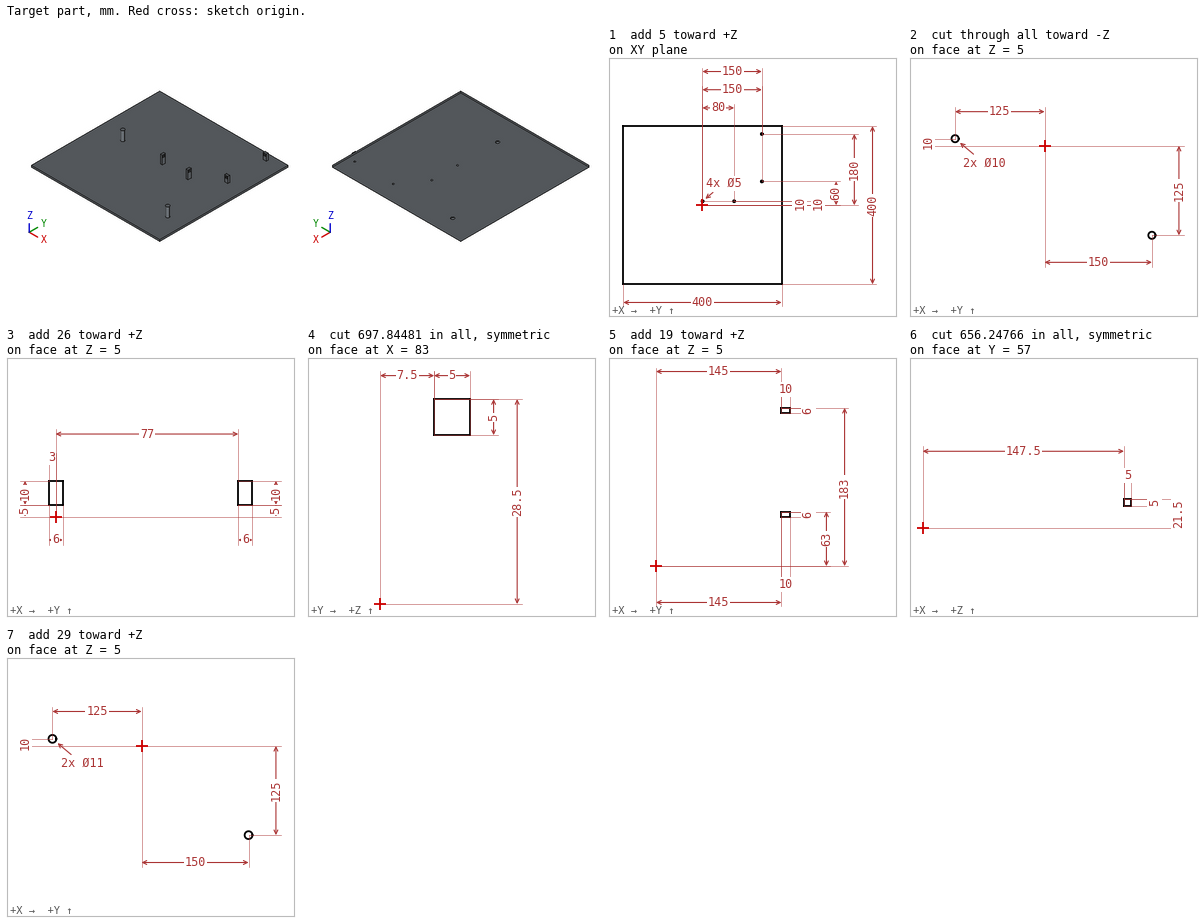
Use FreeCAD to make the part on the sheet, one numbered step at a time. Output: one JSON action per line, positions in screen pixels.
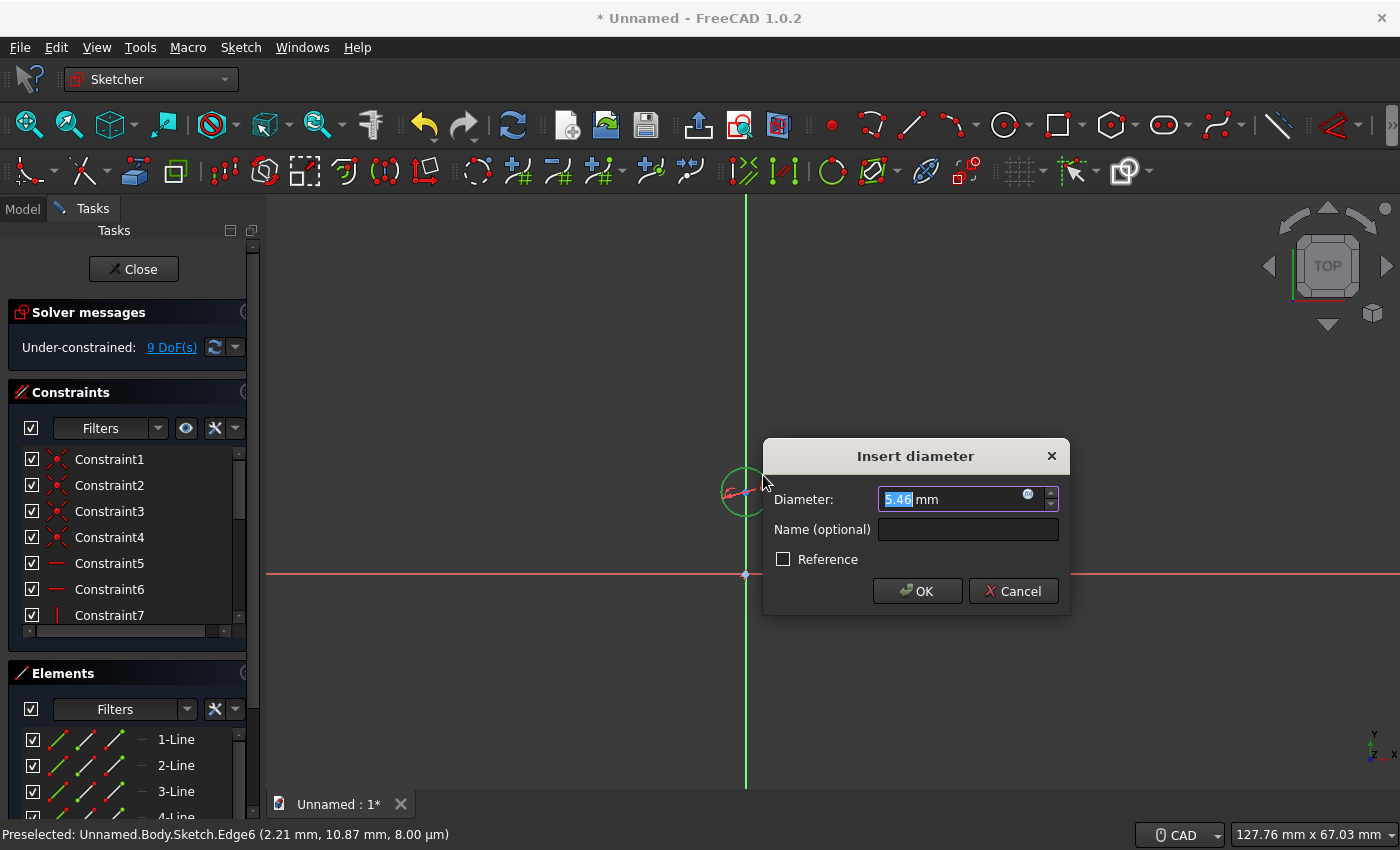
{"action": "type", "text": "5"}
{"action": "key", "text": "Return"}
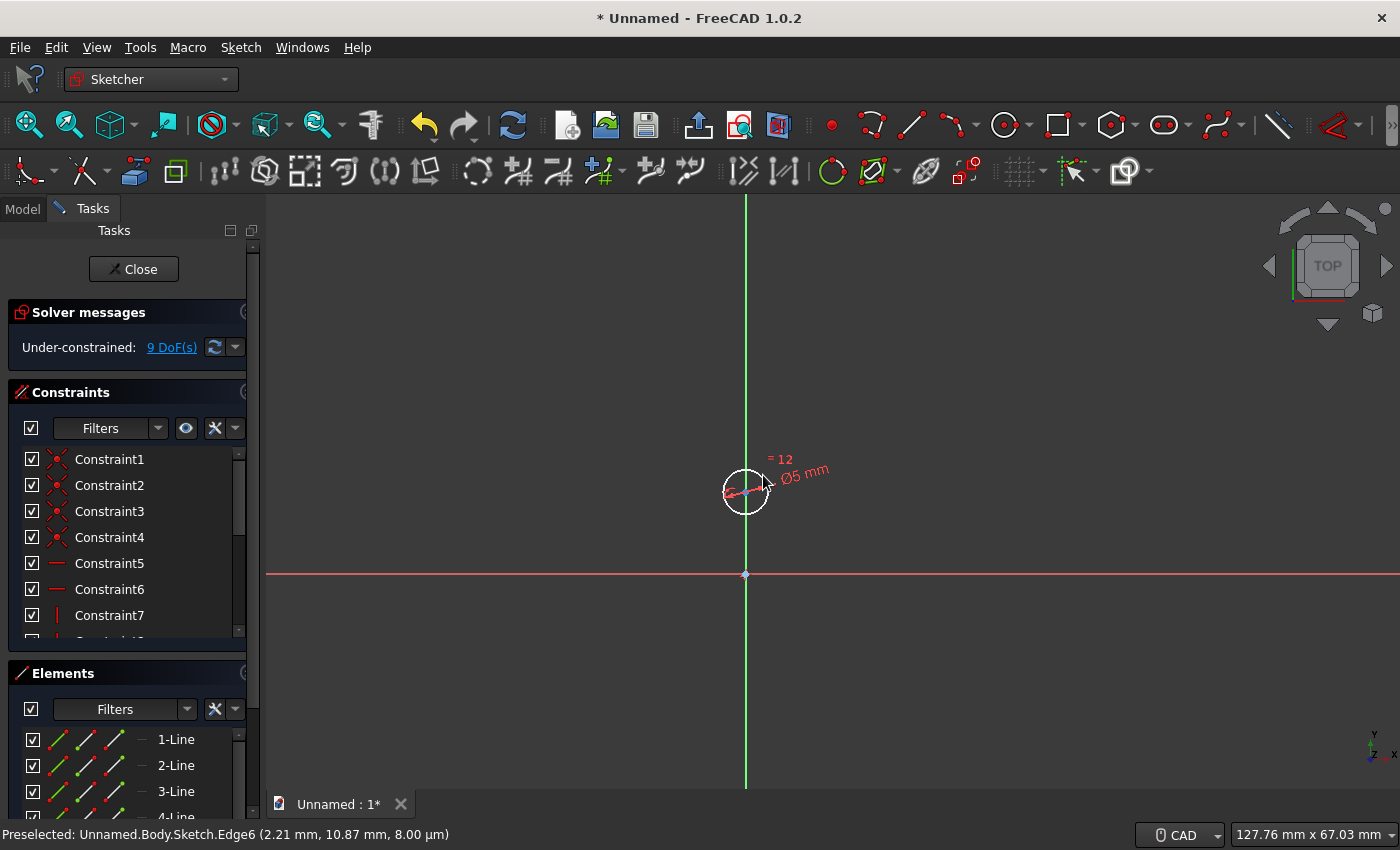
{"action": "left_click", "coordinate": [746, 492]}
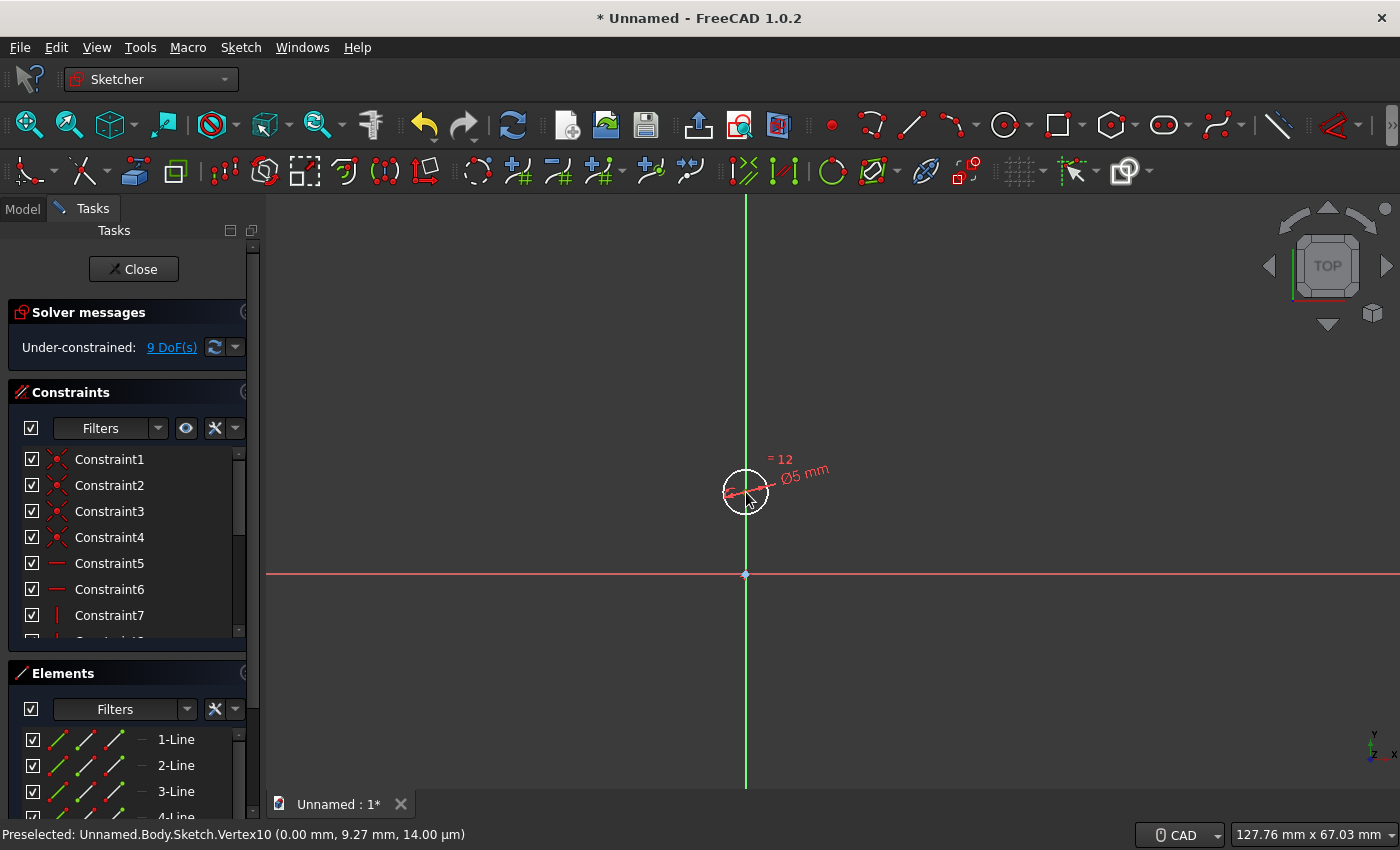
{"action": "key", "text": "i"}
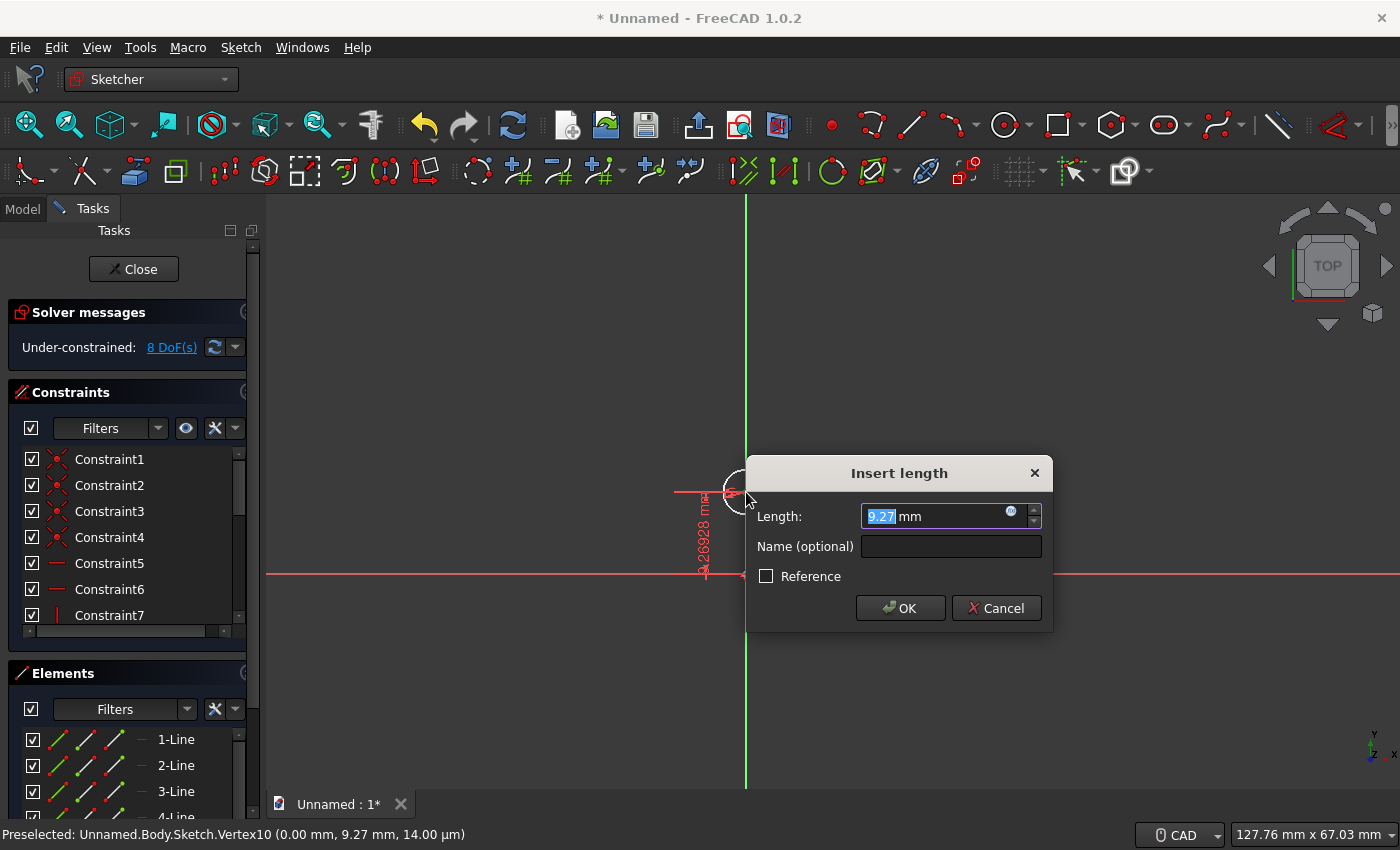
{"action": "type", "text": "10"}
{"action": "key", "text": "Return"}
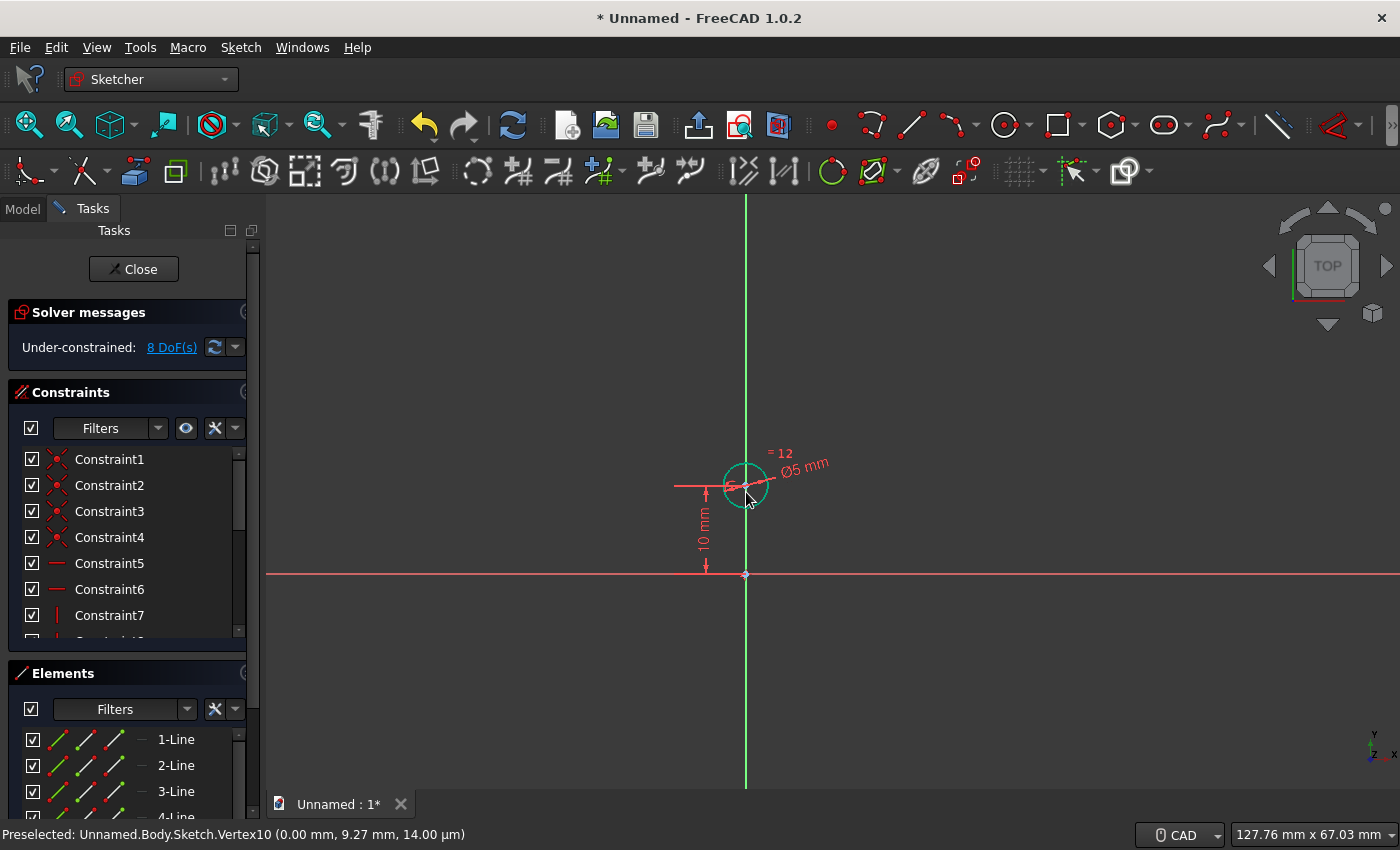
{"action": "scroll", "coordinate": [767, 481], "scroll_direction": "down", "scroll_amount": 11}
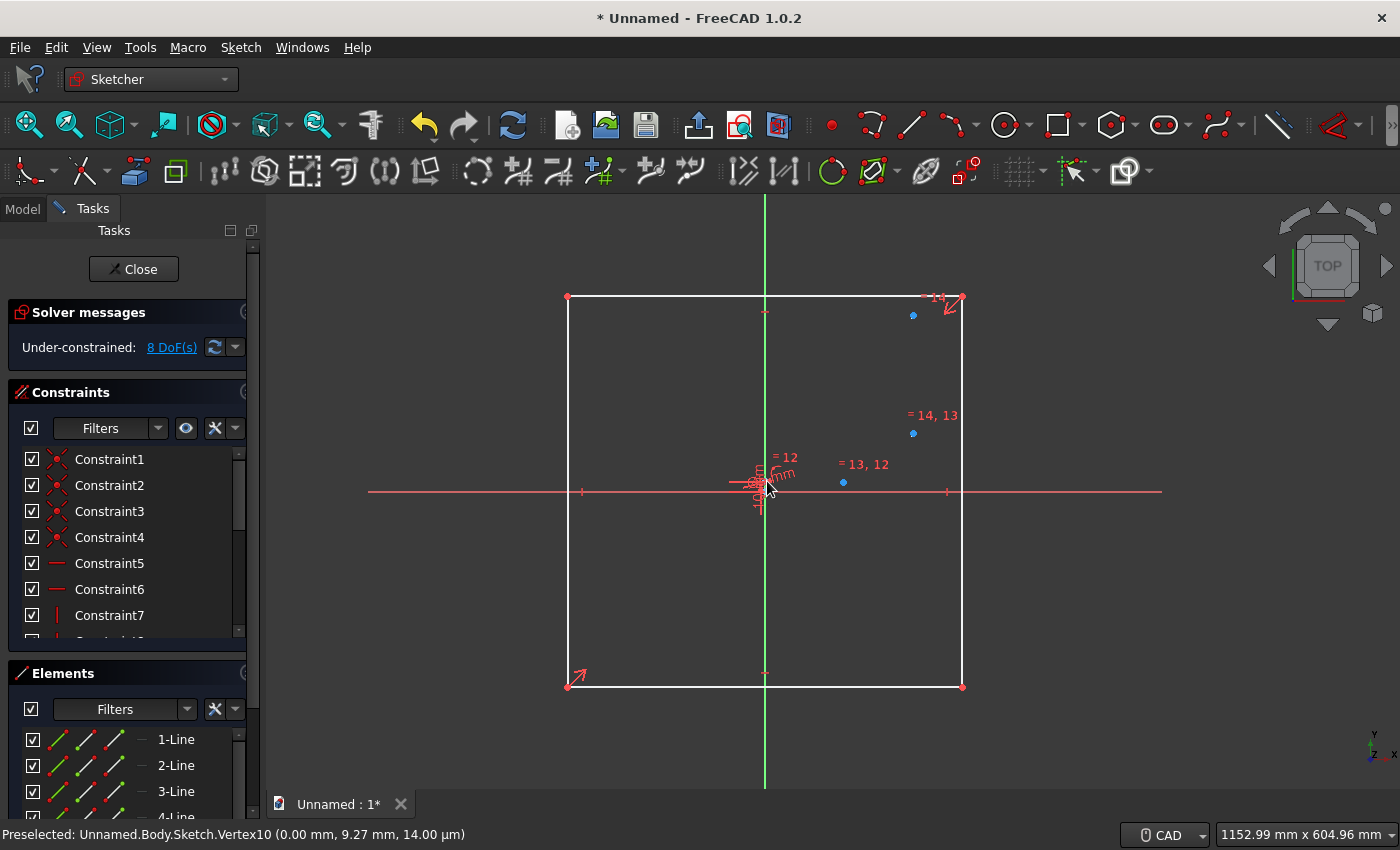
{"action": "left_click", "coordinate": [844, 483]}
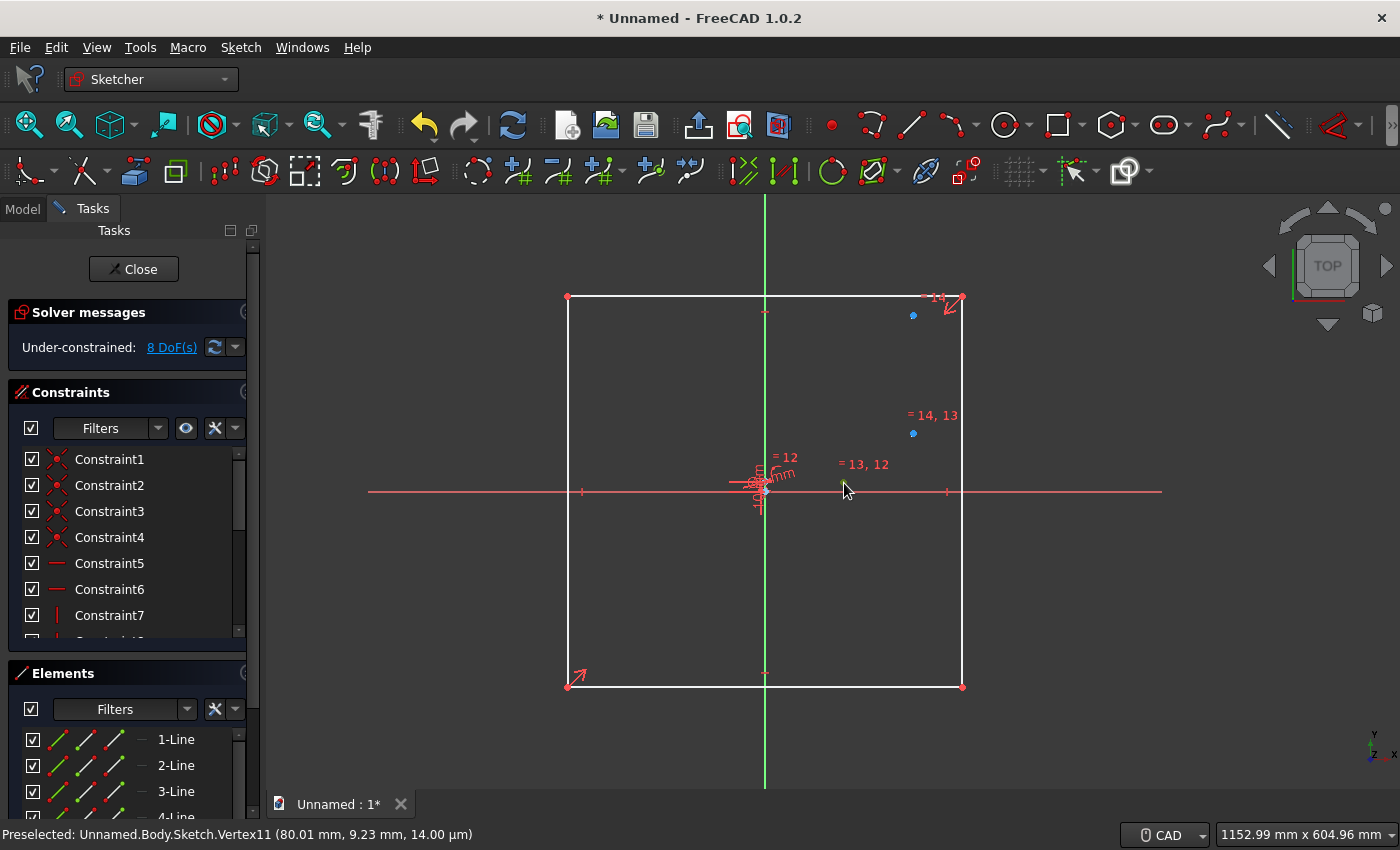
{"action": "key", "text": "l"}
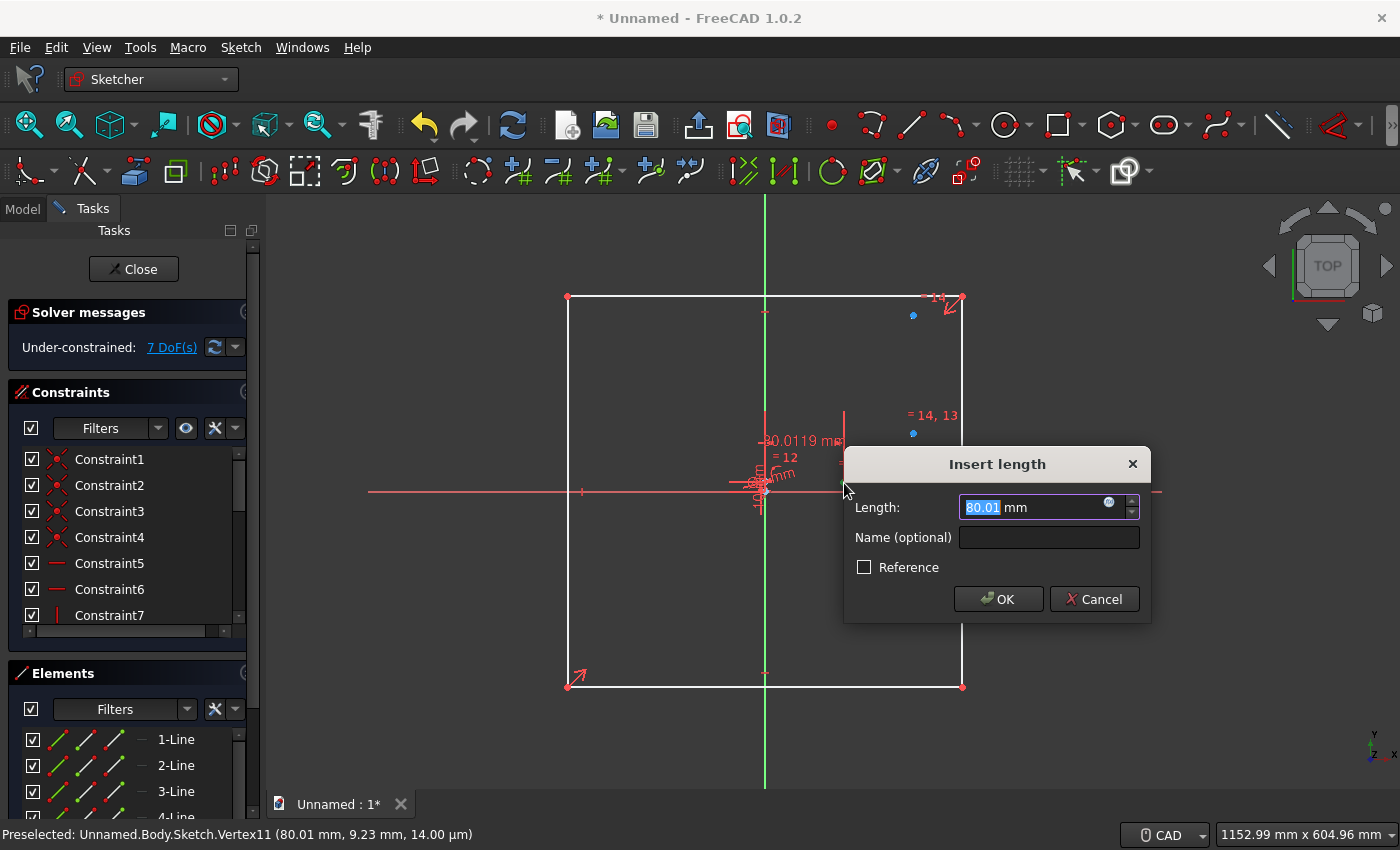
{"action": "type", "text": "80"}
{"action": "key", "text": "Return"}